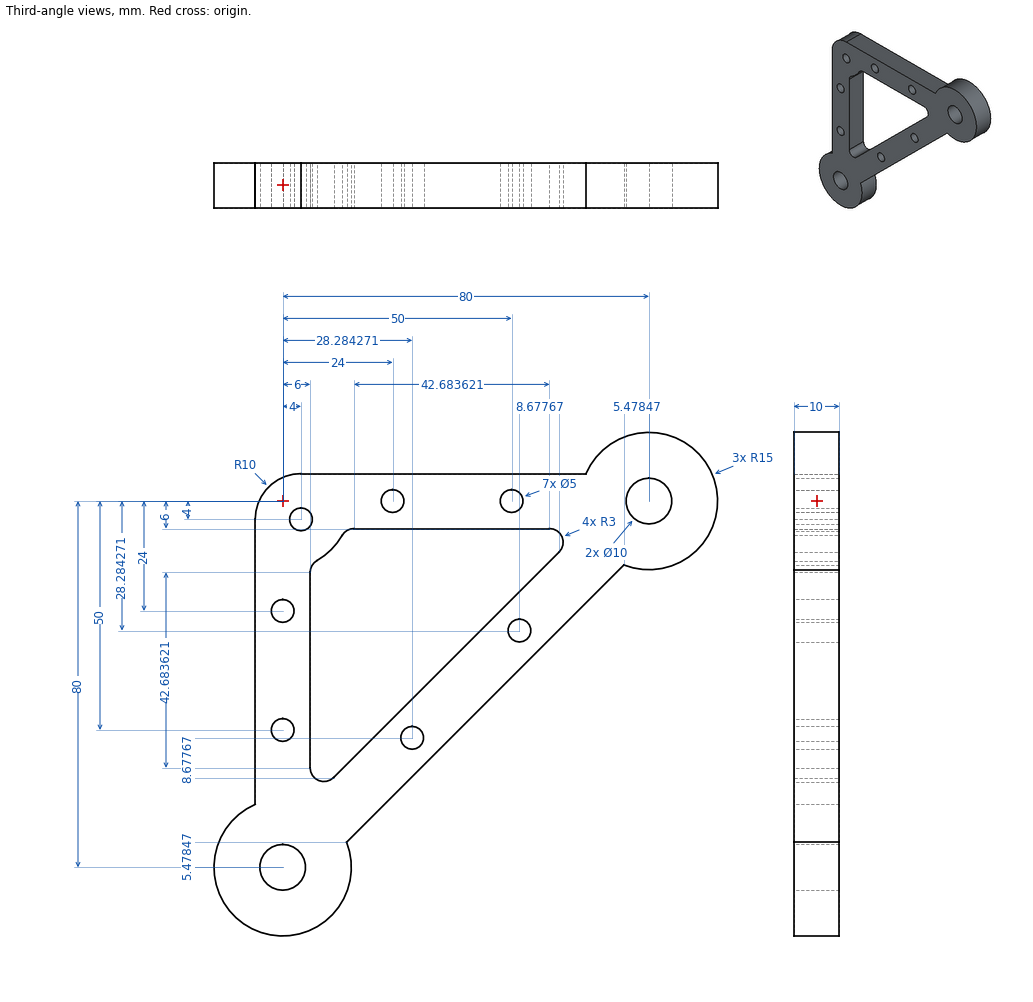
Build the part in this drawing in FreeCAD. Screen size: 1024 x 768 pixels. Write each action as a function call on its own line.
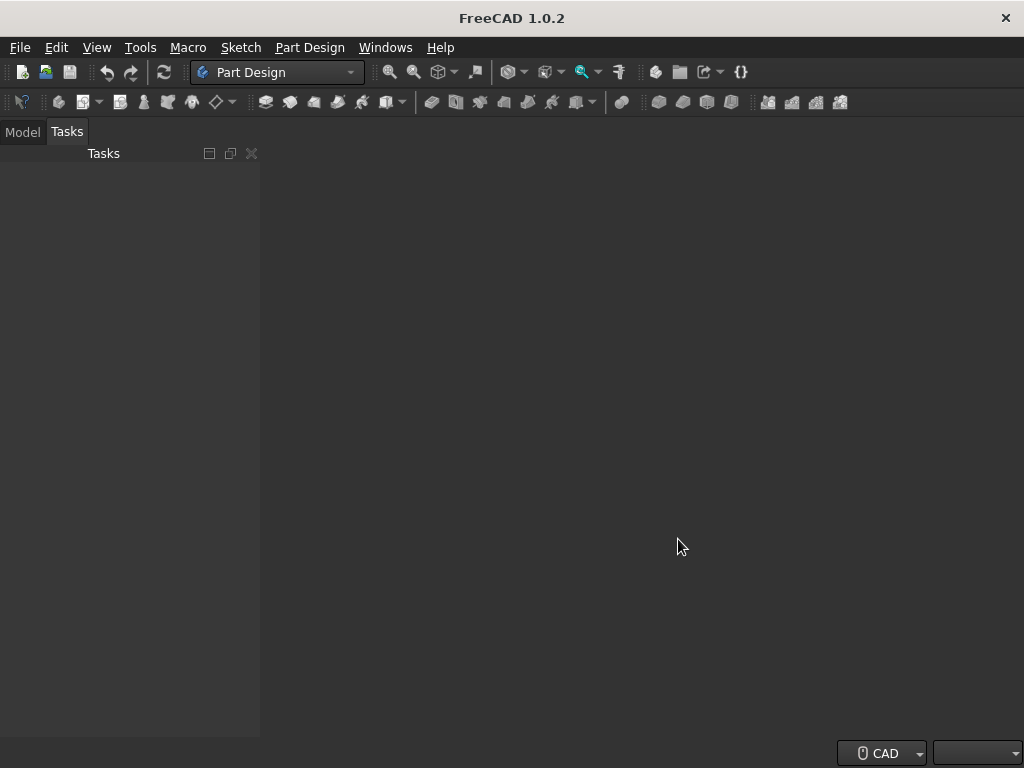
key(ctrl+n)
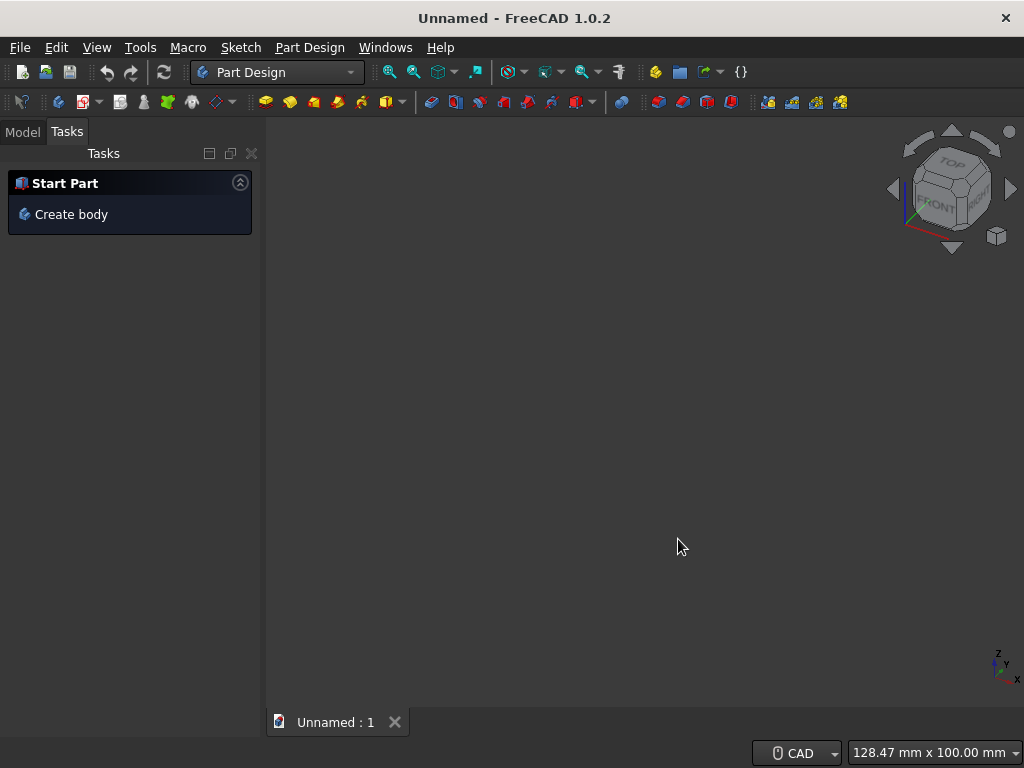
click(84, 102)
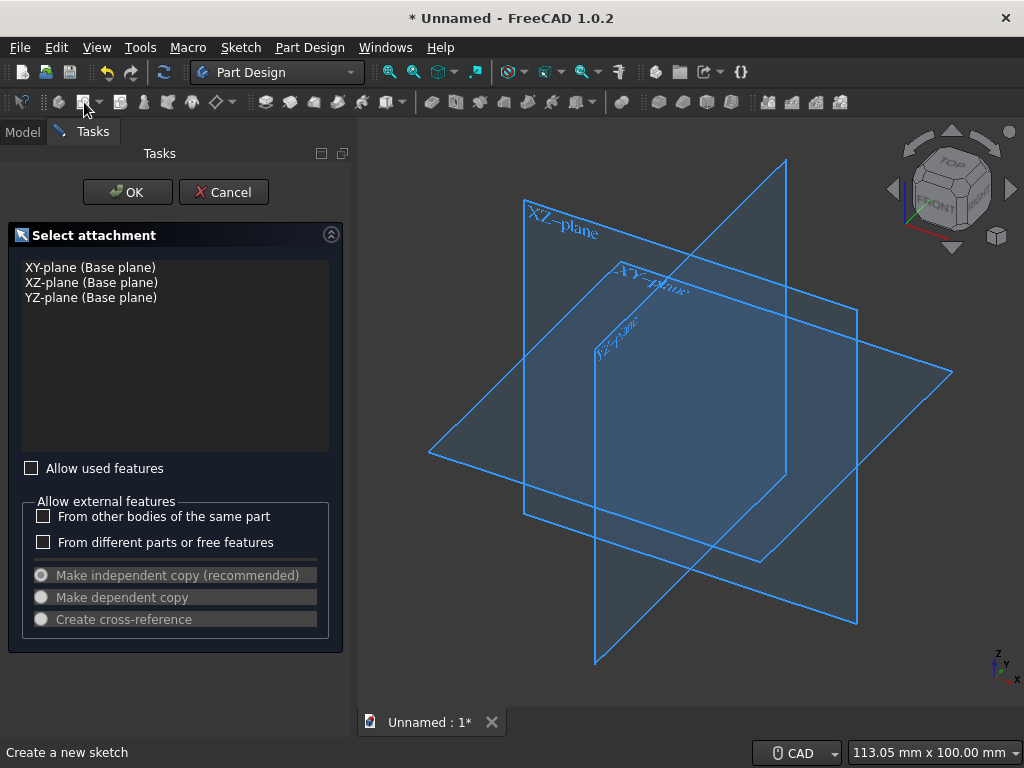
click(82, 282)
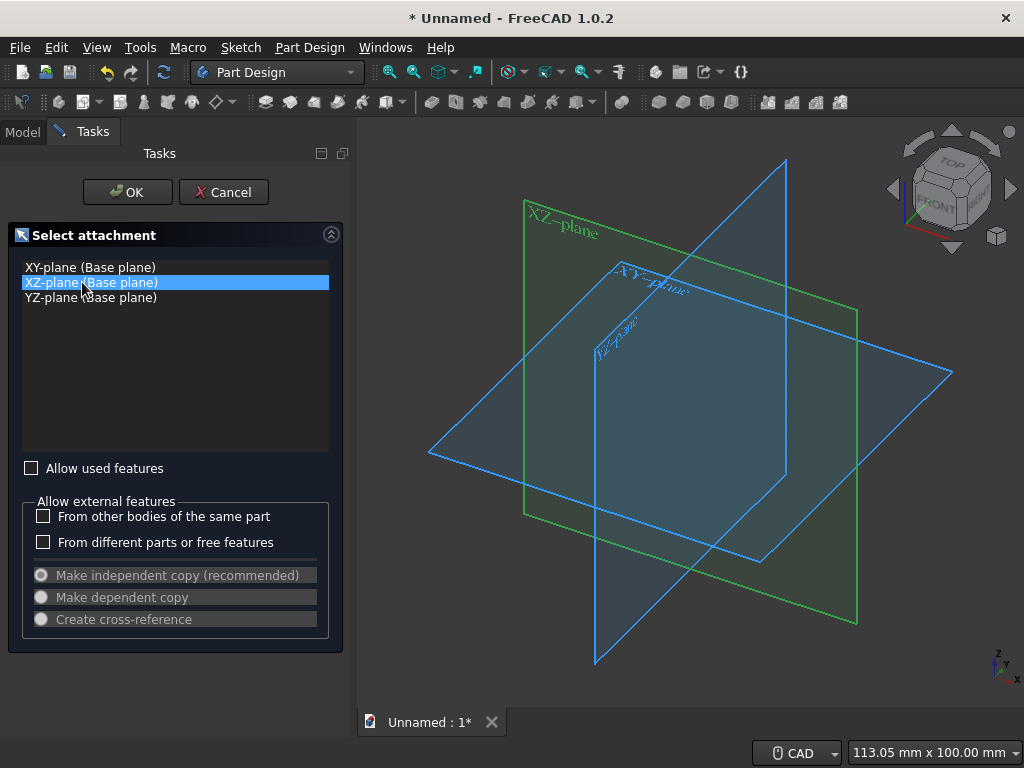
click(128, 192)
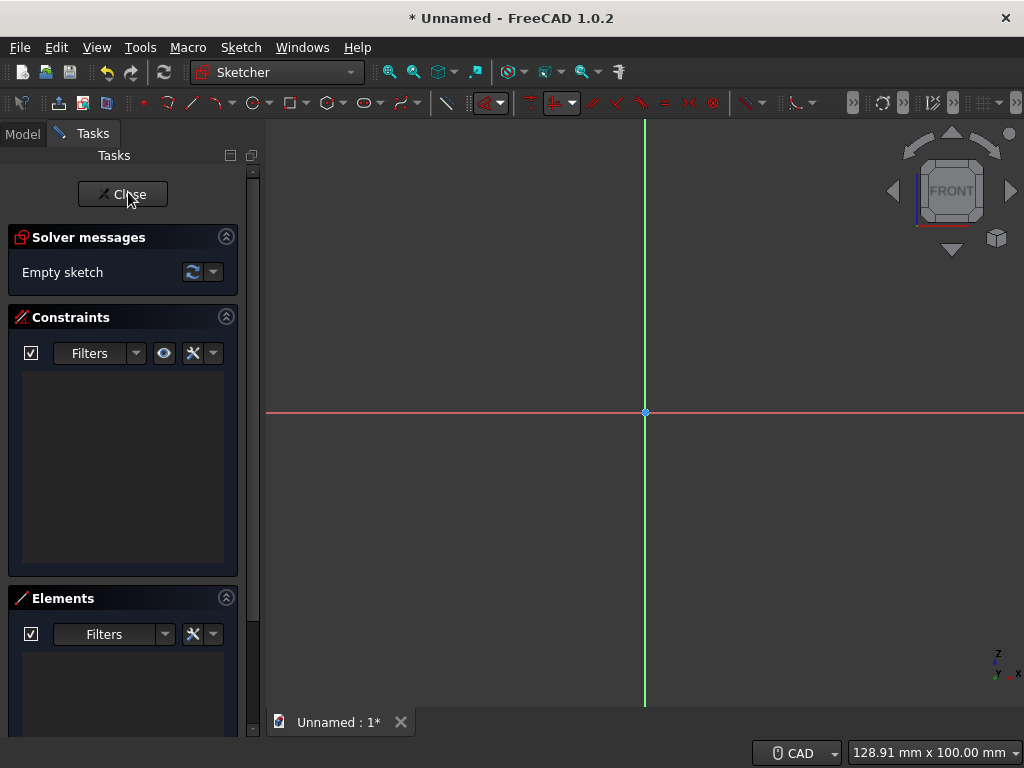
scroll(294, 147, down, 3)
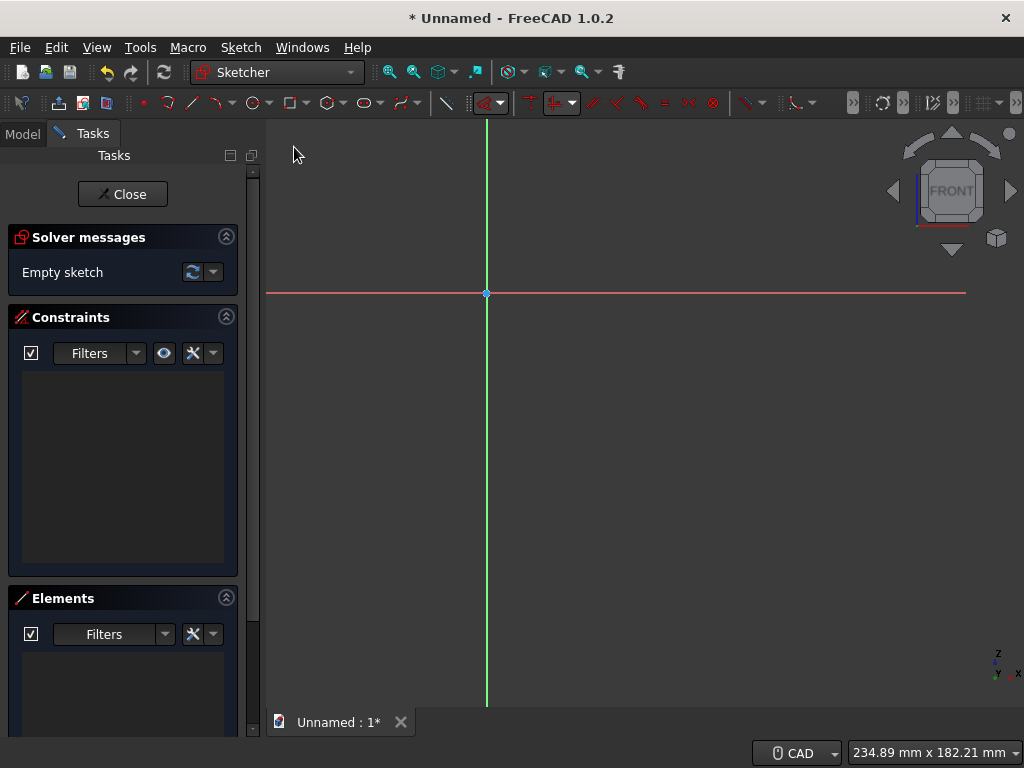
click(192, 104)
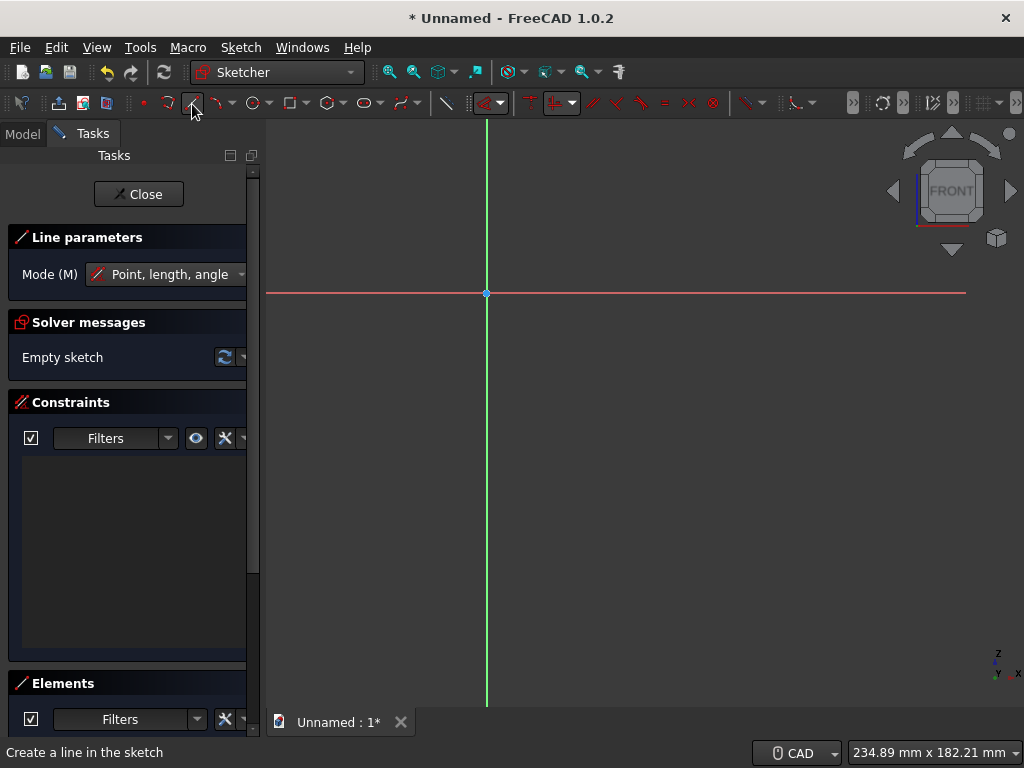
click(467, 507)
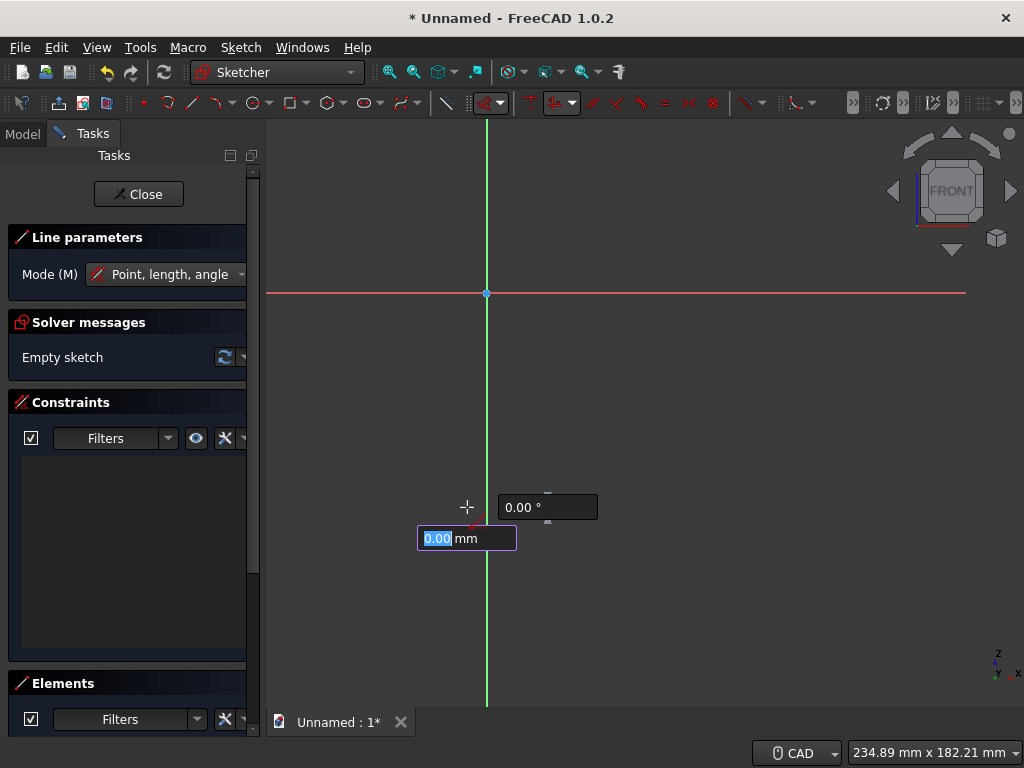
scroll(467, 306, up, 2)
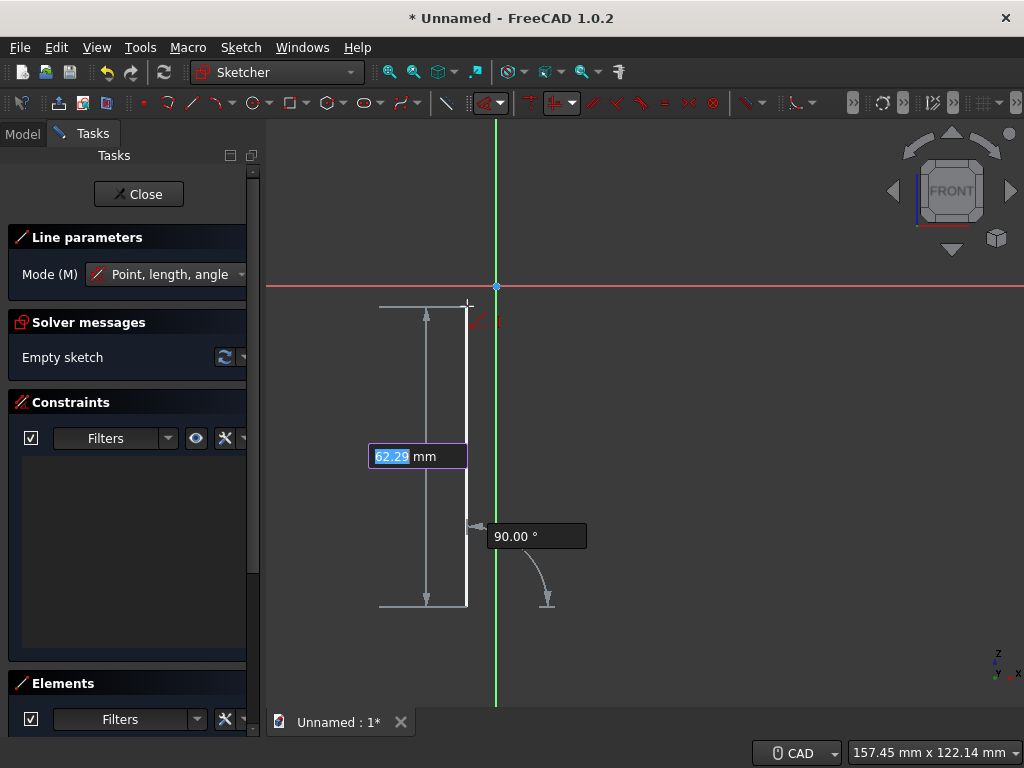
click(467, 306)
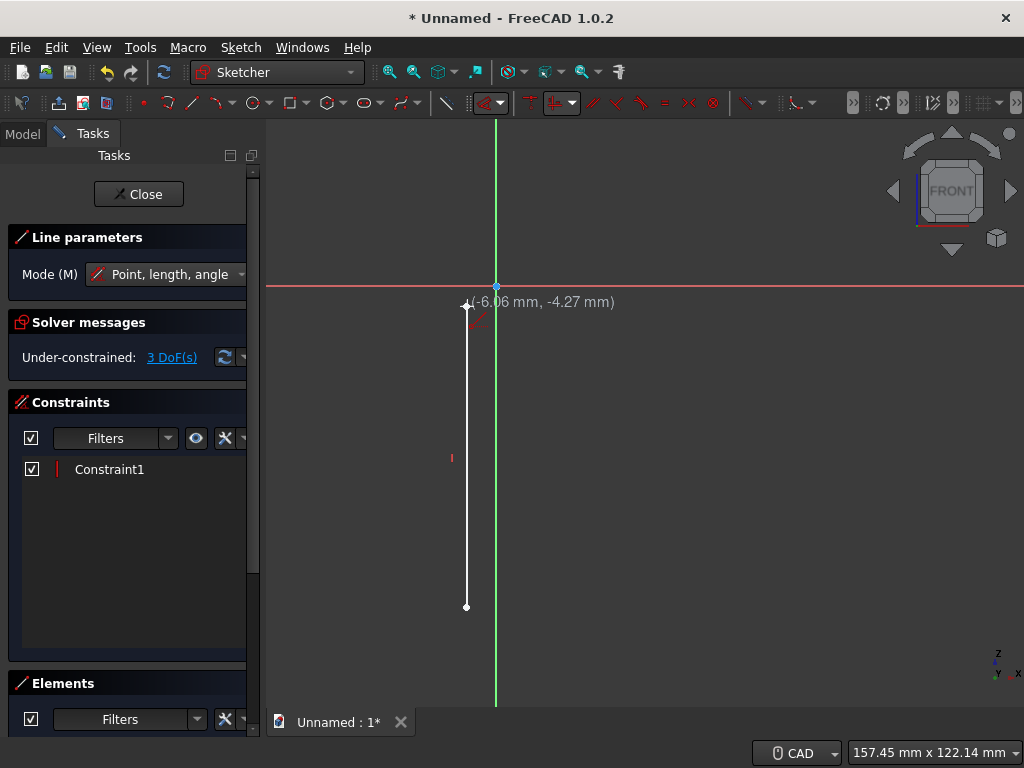
click(515, 258)
click(815, 258)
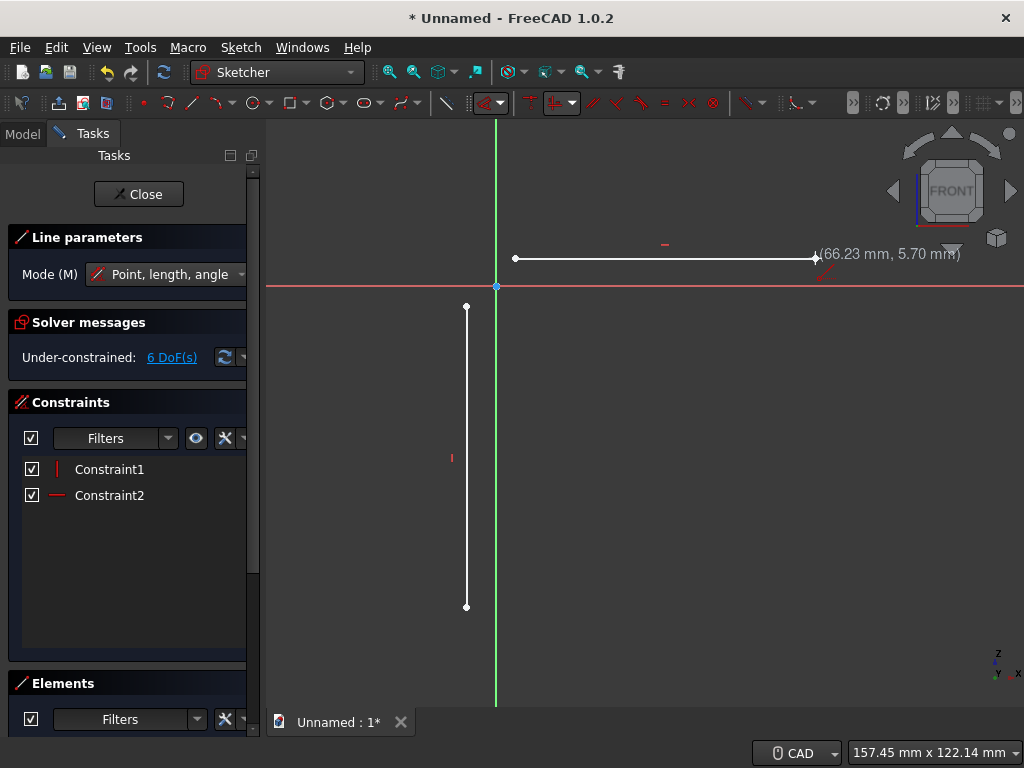
click(855, 354)
click(563, 645)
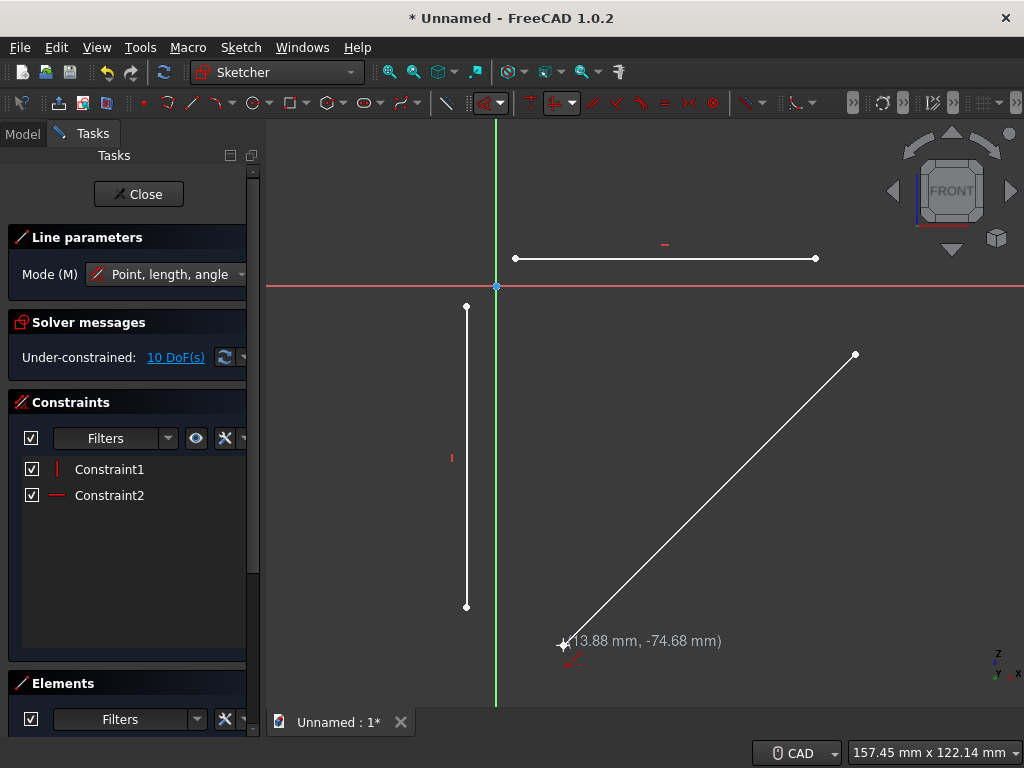
key(g)
key(3)
key(a)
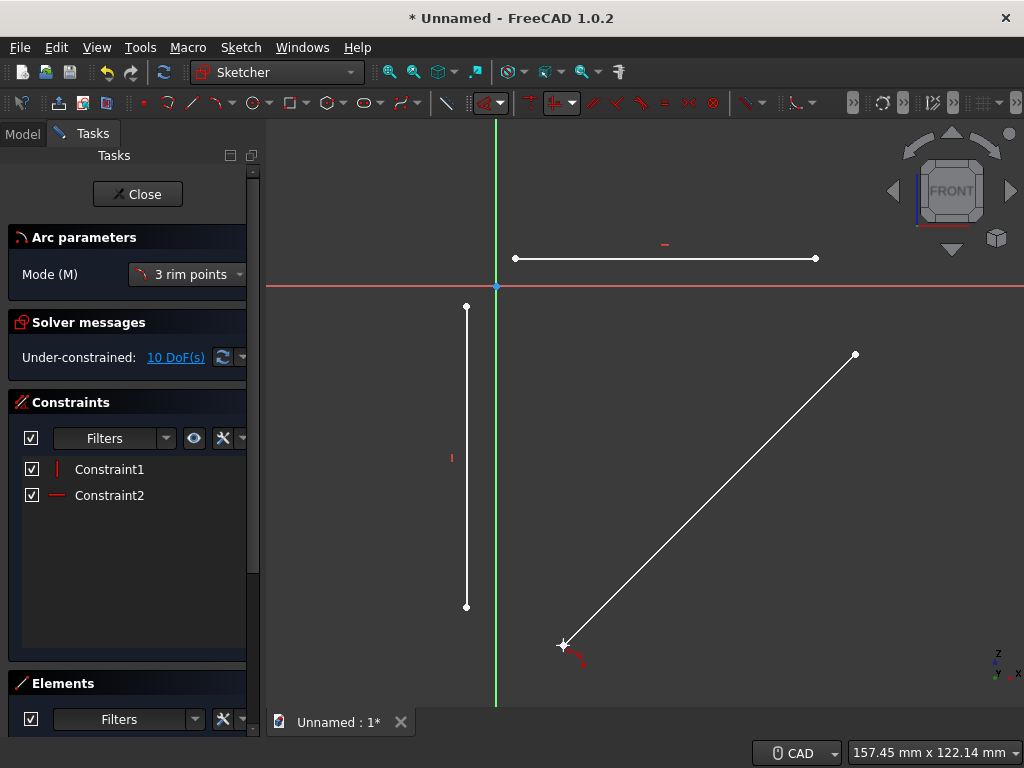
click(467, 307)
click(515, 259)
click(481, 272)